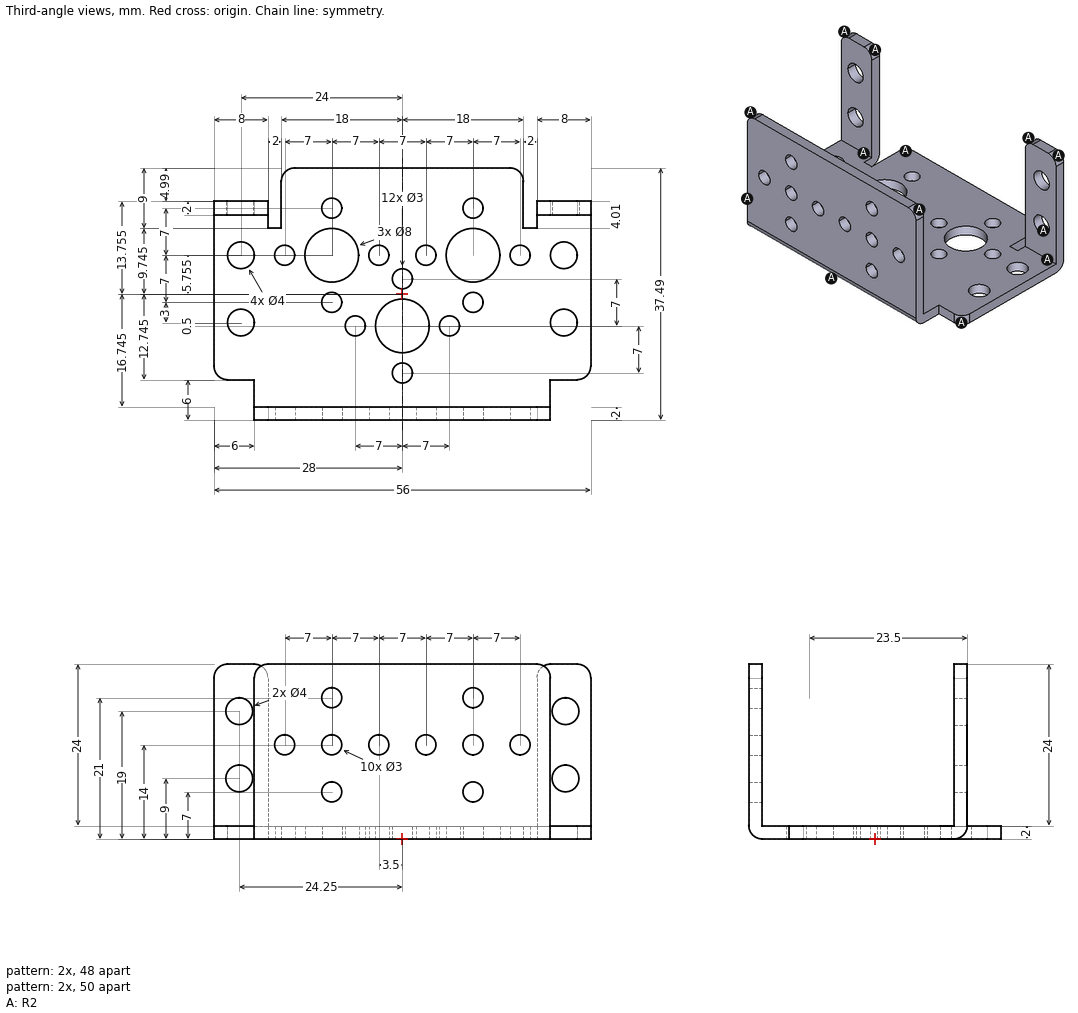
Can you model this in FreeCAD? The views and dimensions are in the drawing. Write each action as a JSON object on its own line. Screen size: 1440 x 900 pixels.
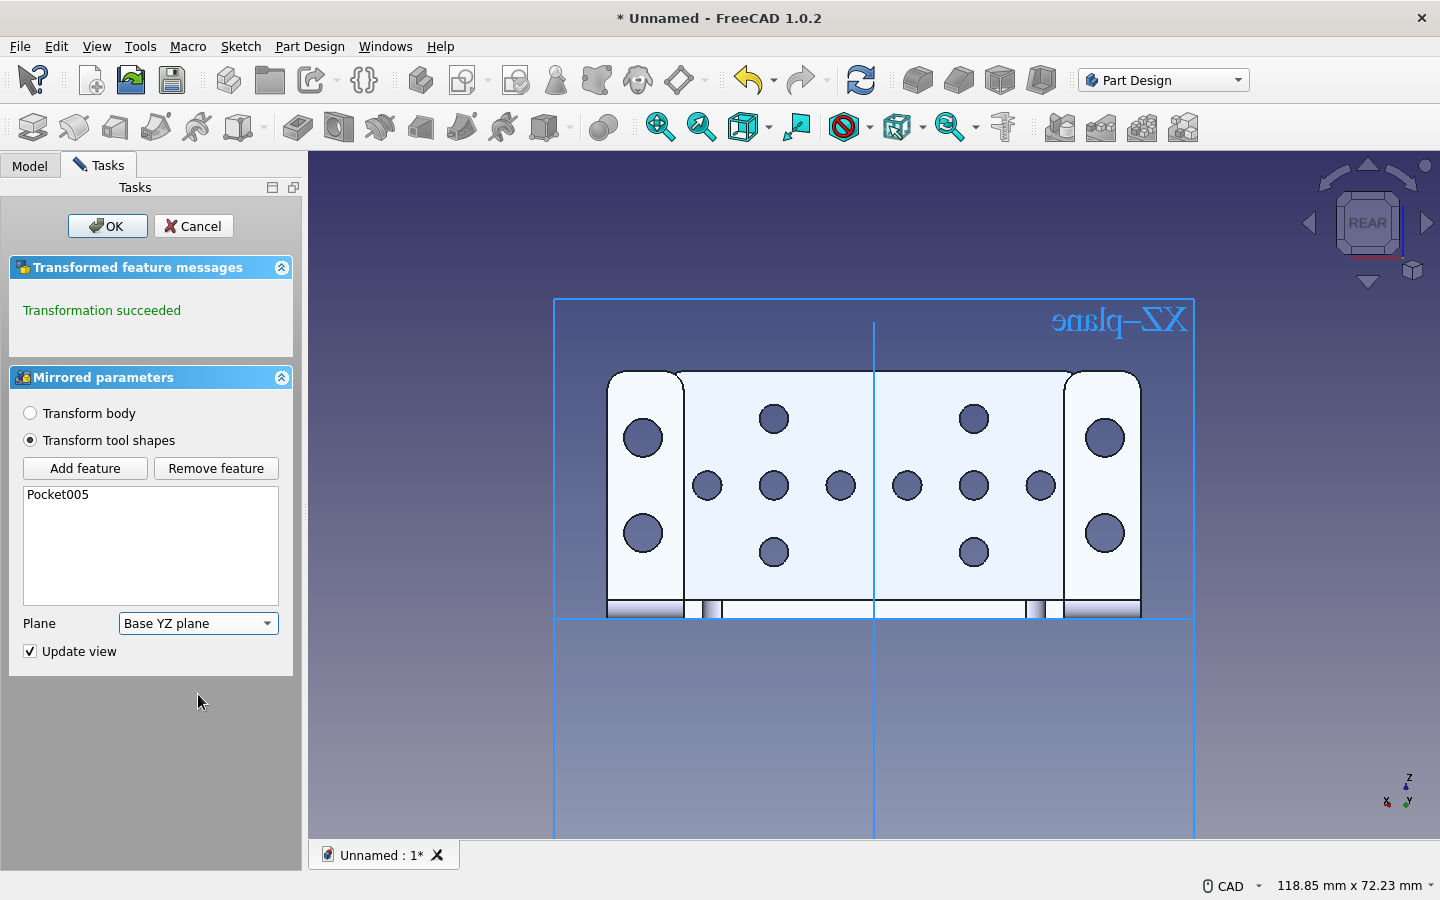
{"action": "left_click", "coordinate": [108, 226]}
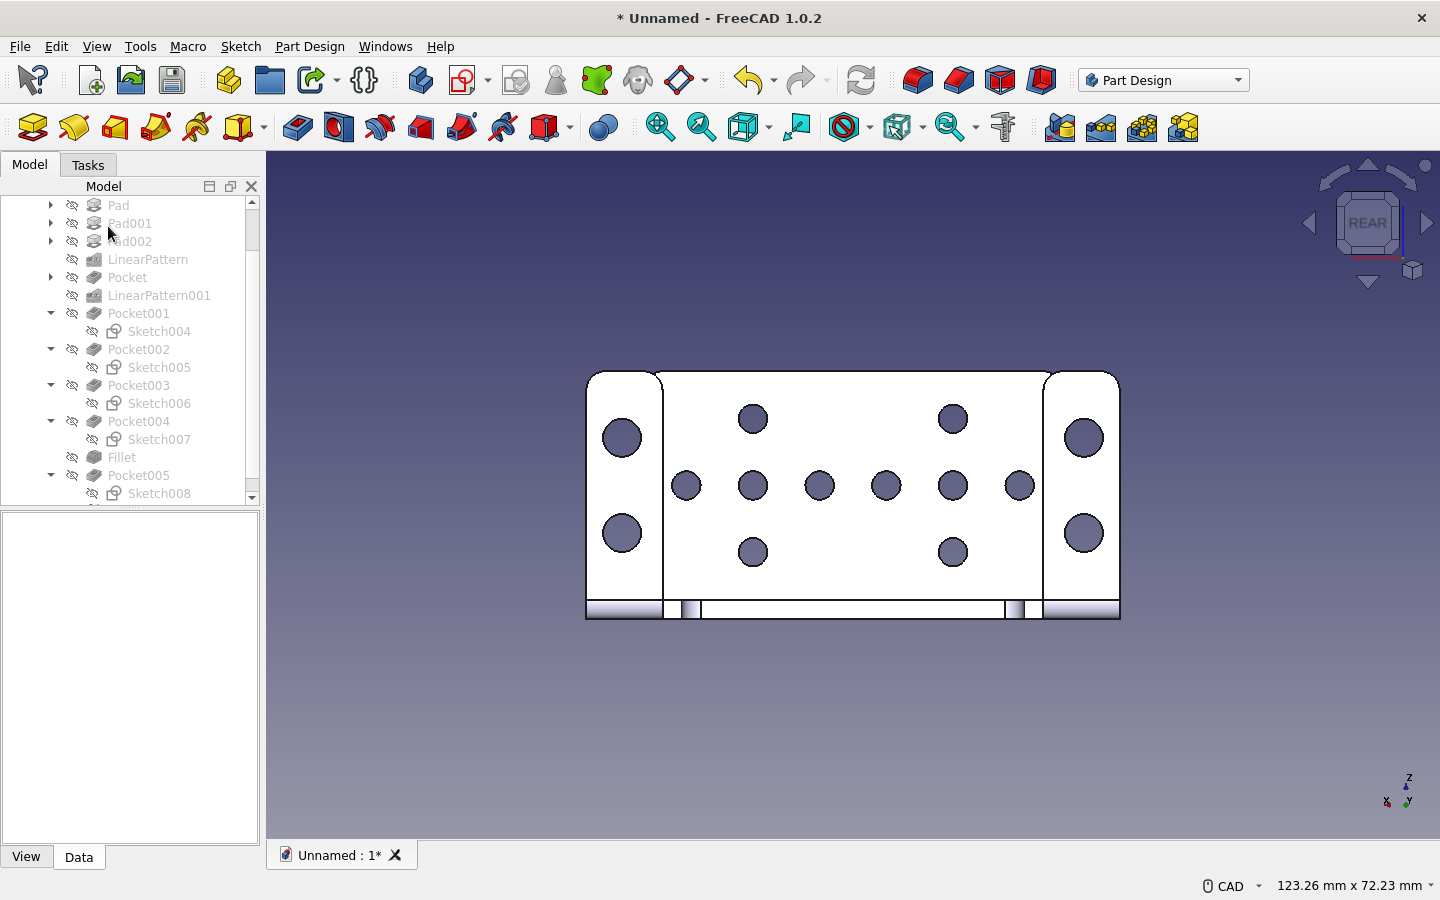
{"action": "key", "text": "0"}